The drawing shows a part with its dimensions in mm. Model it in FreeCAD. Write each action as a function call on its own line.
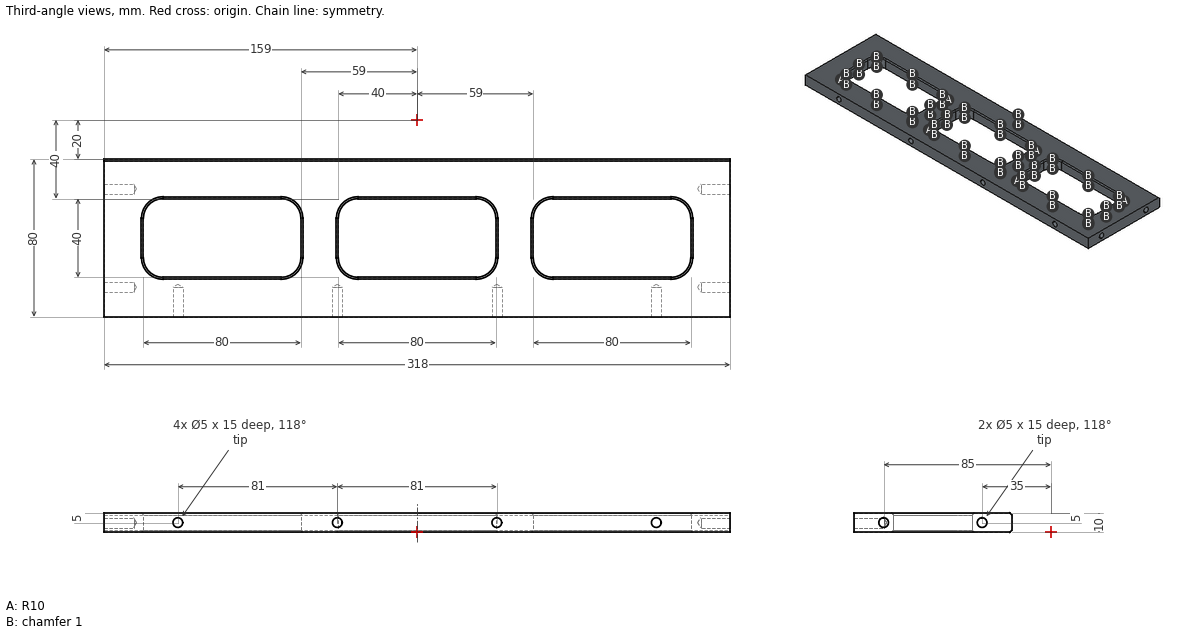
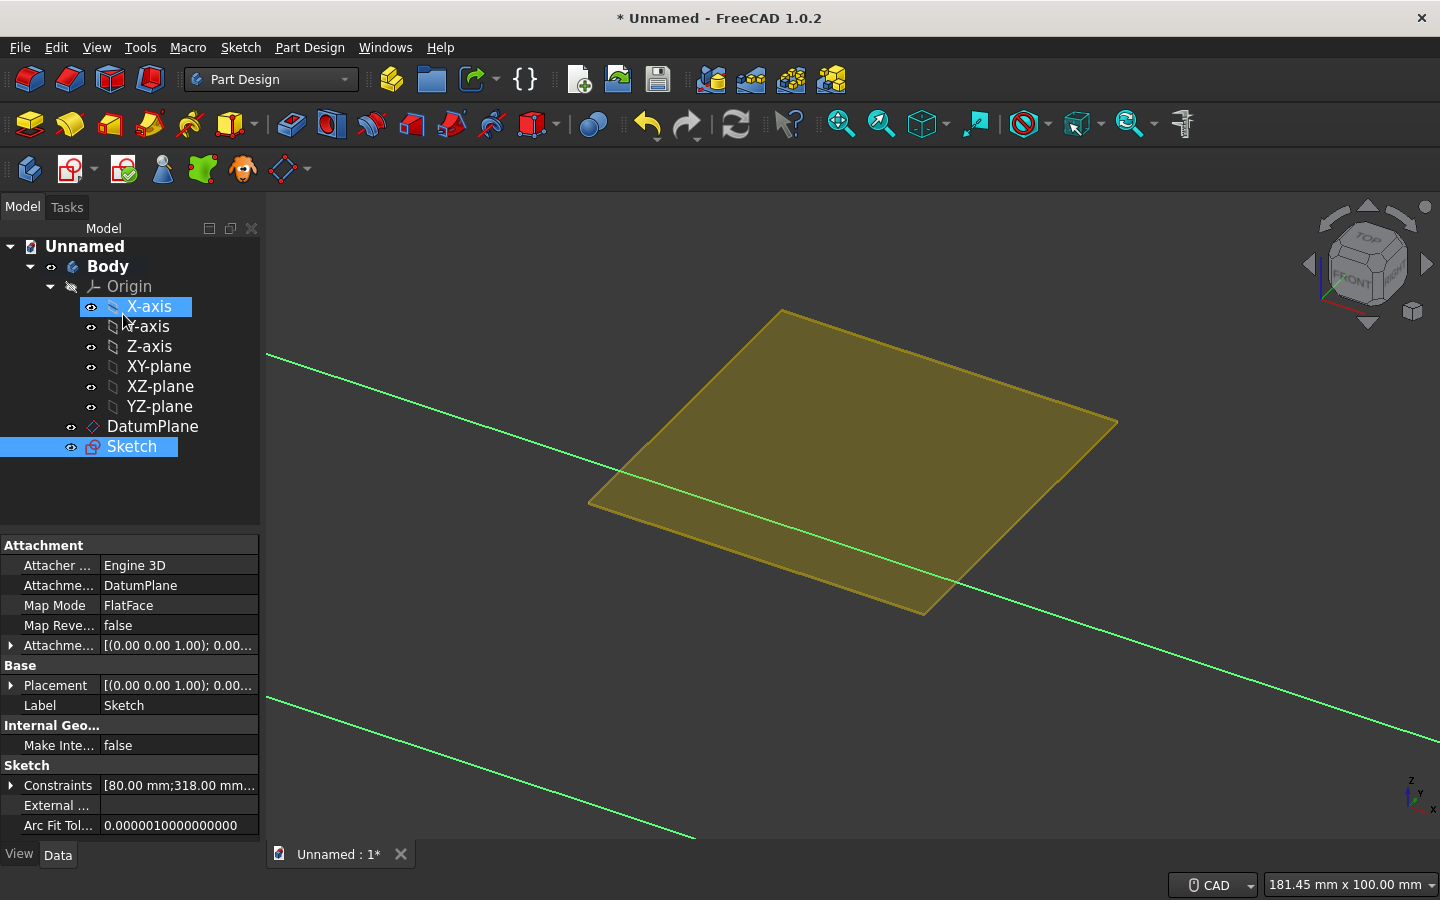
click(30, 124)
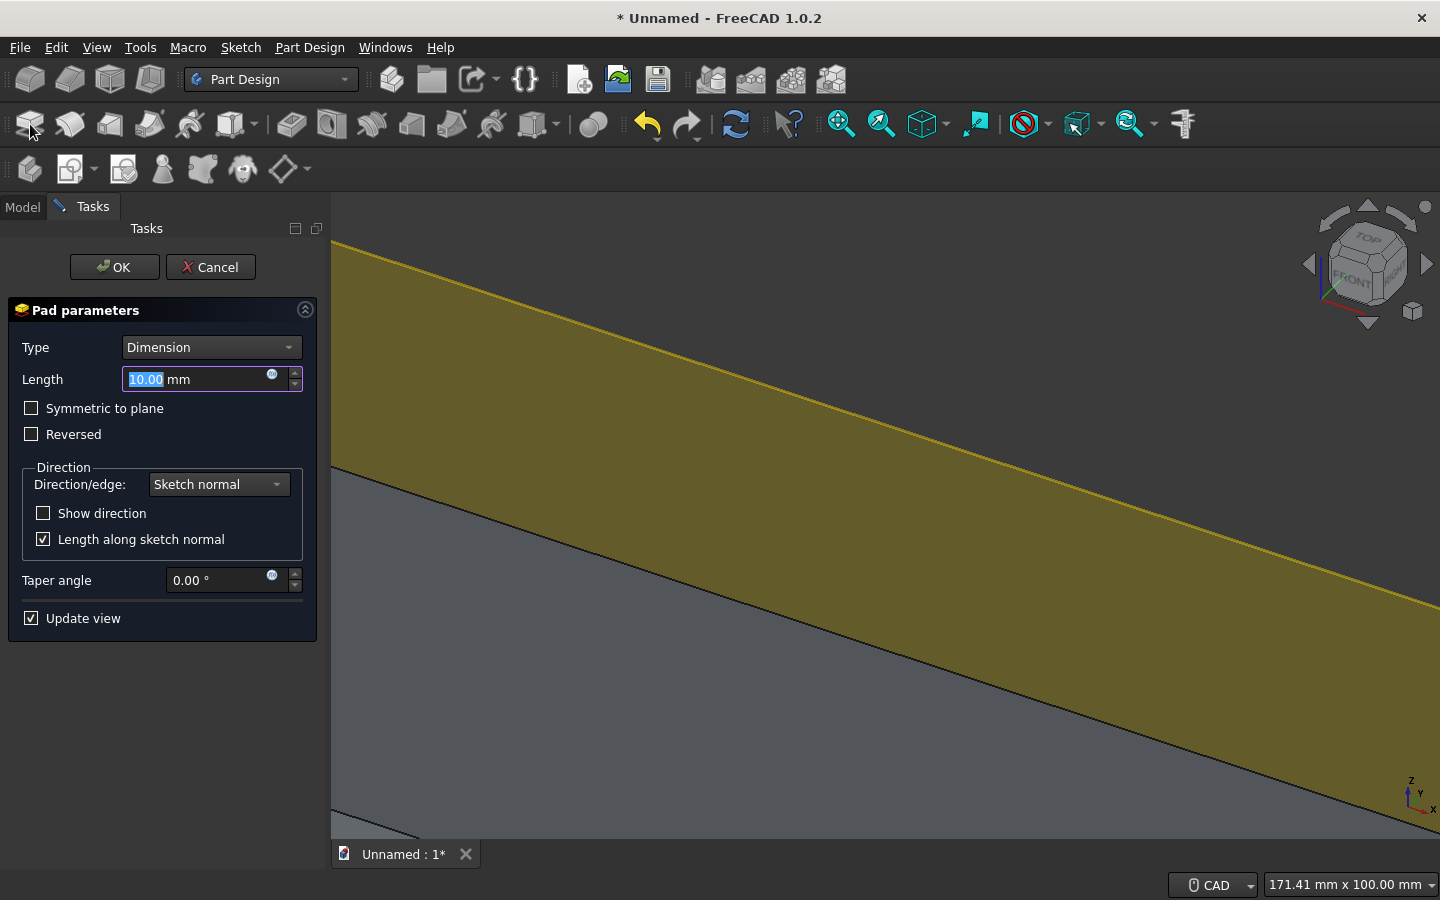
text(10)
key(Tab)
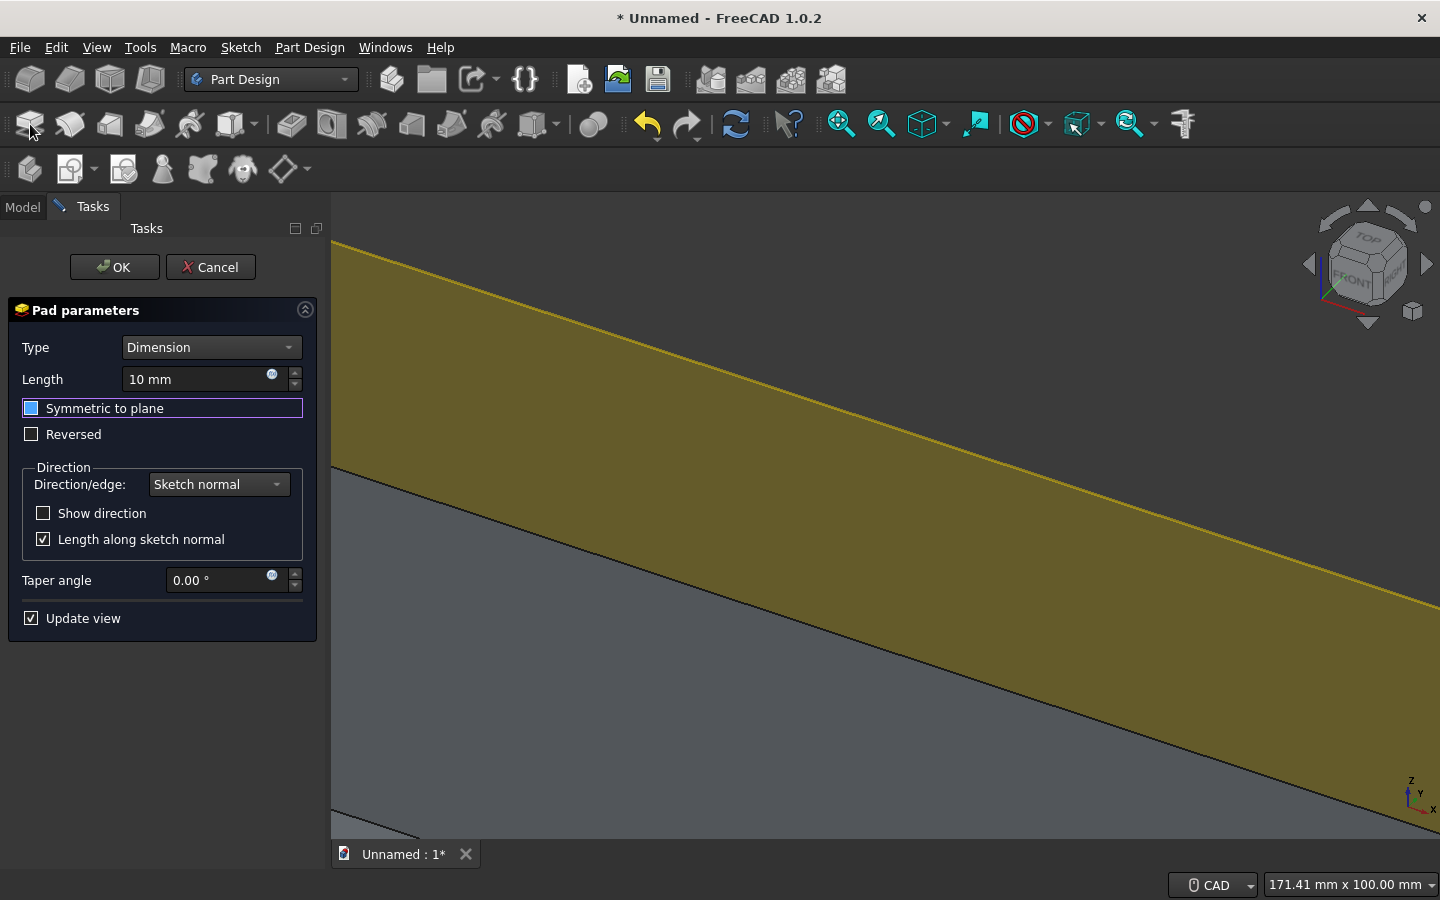
click(30, 434)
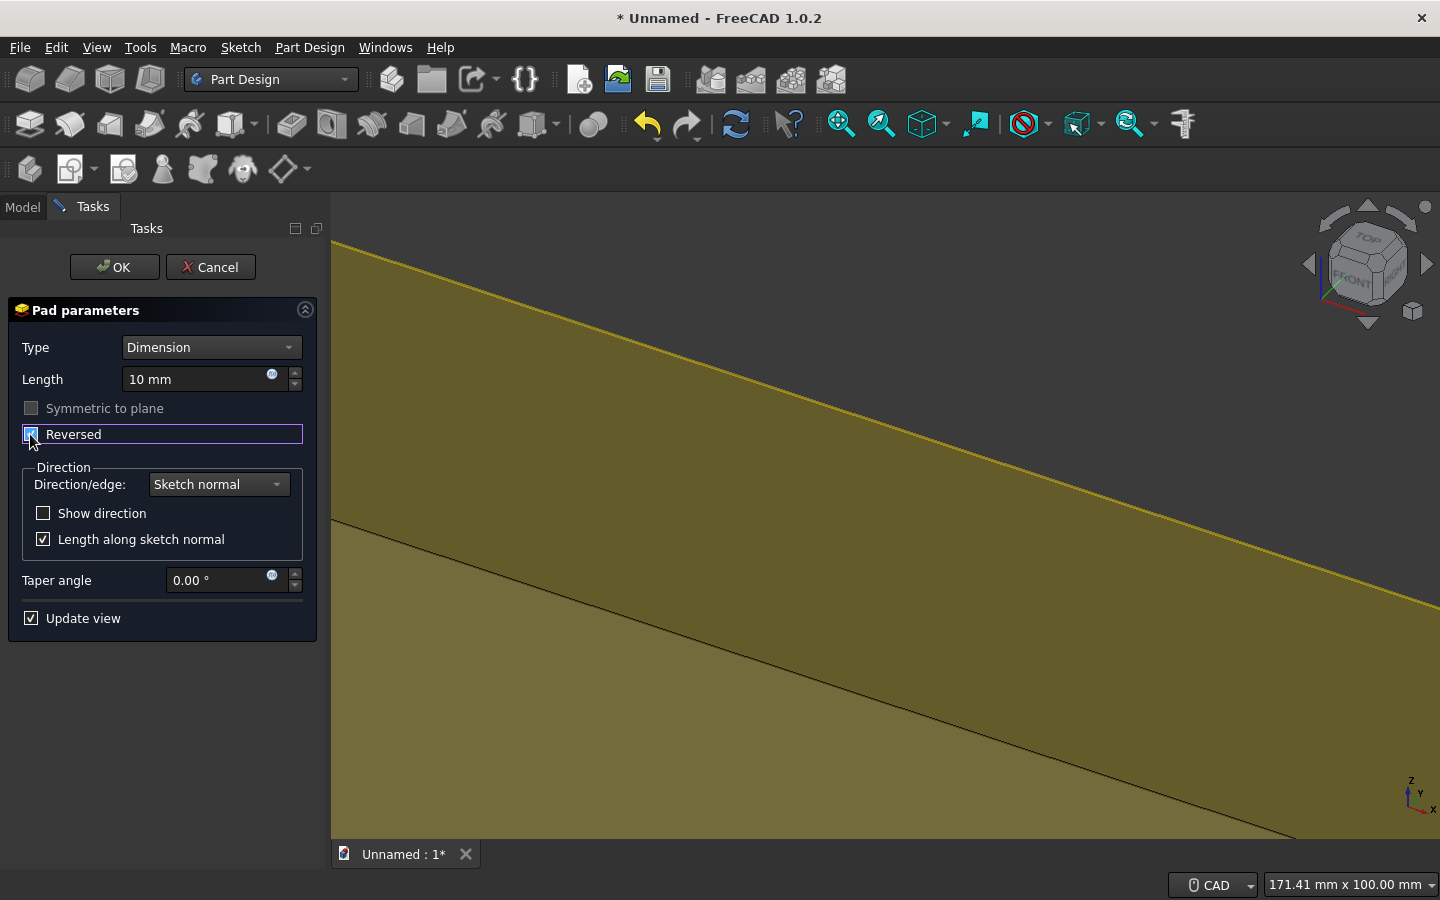
click(115, 267)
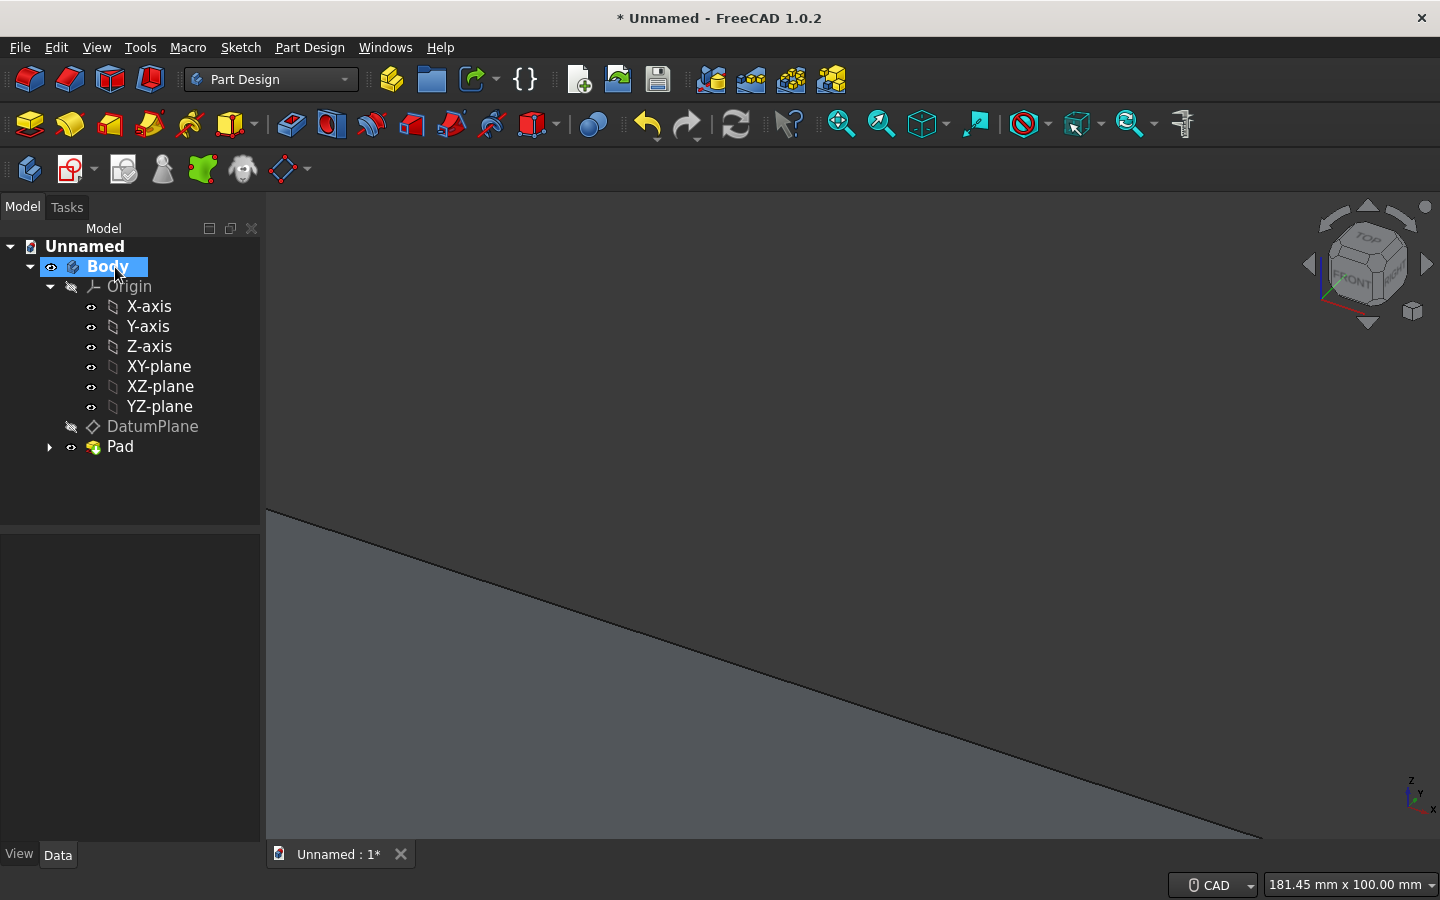
click(842, 124)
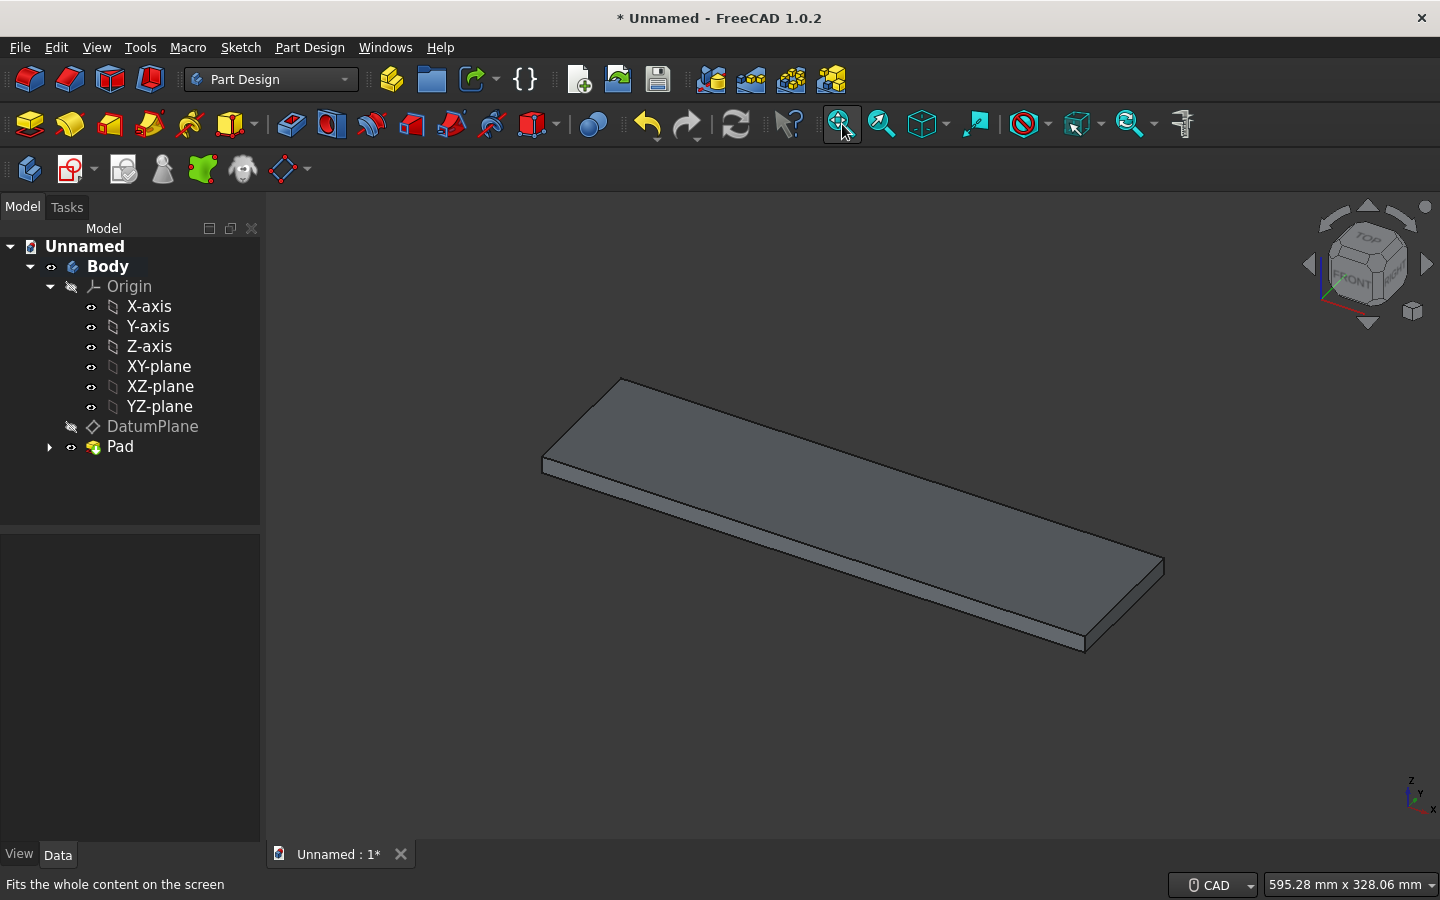
click(1008, 558)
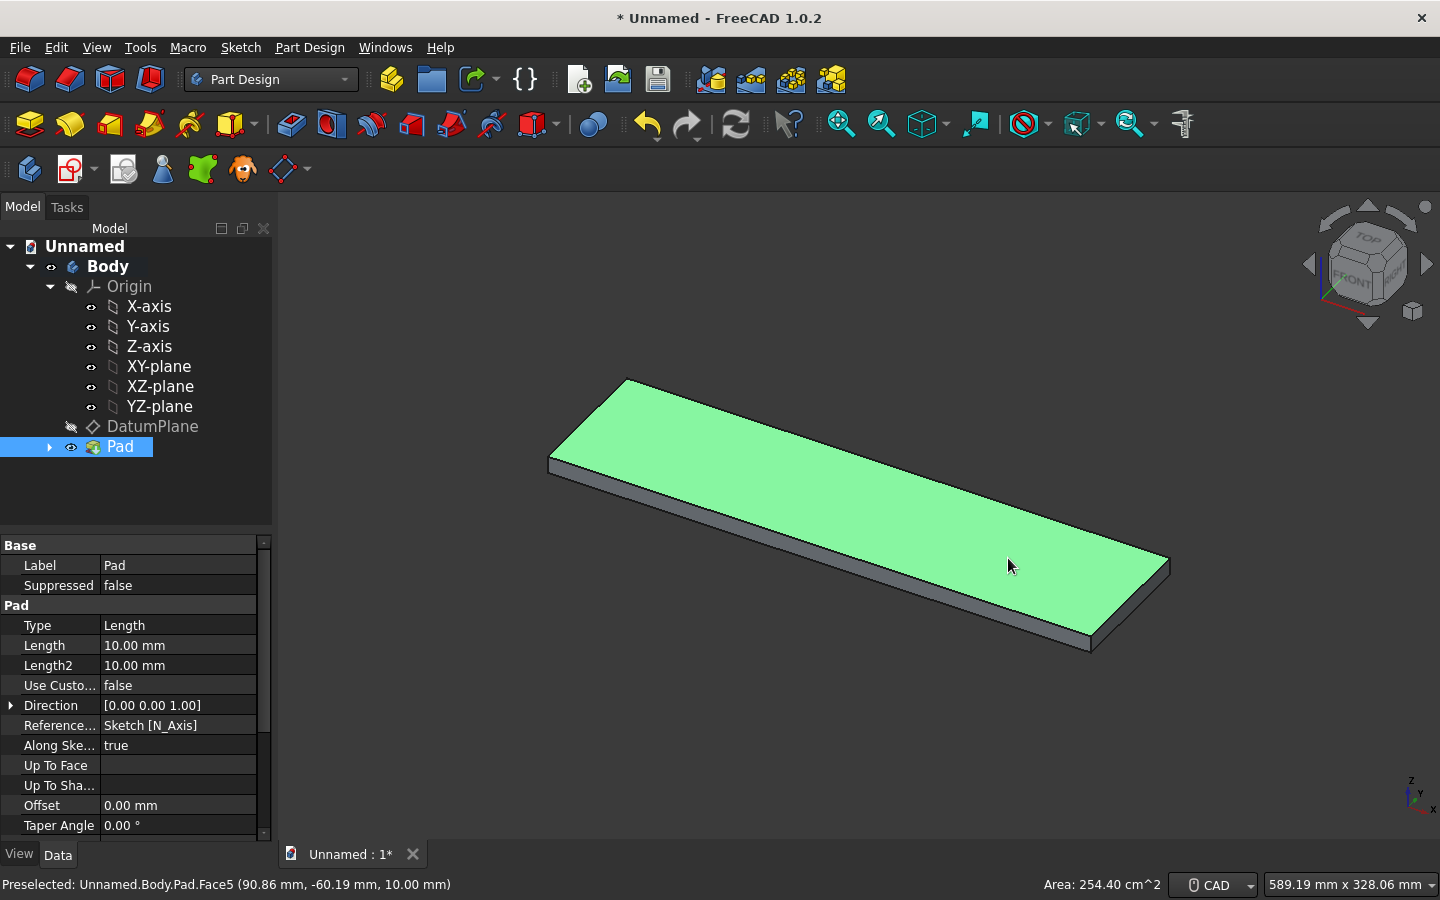
click(70, 170)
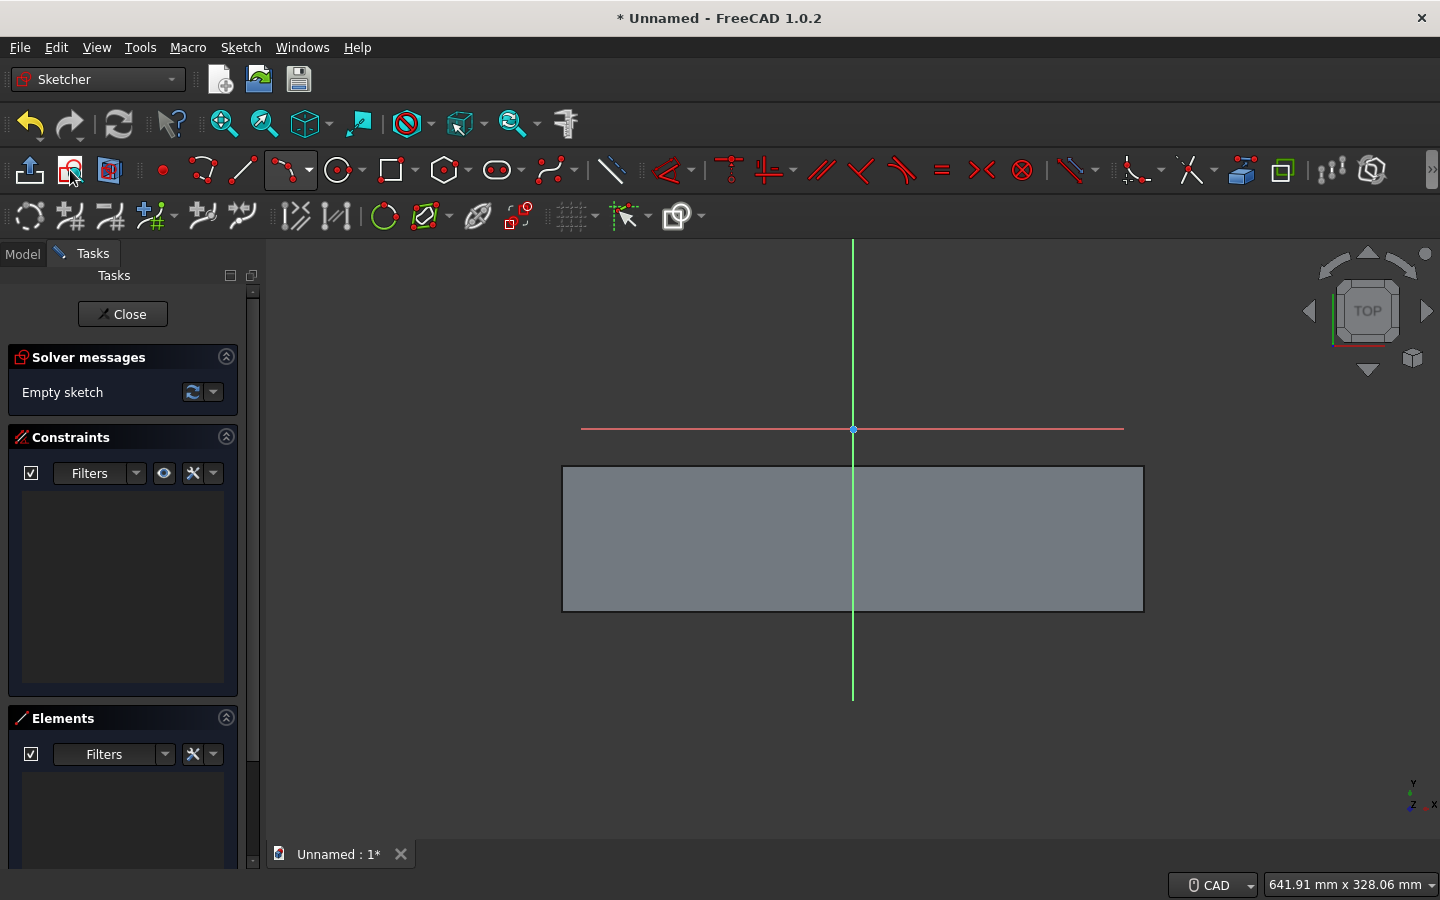
scroll(893, 481, up, 5)